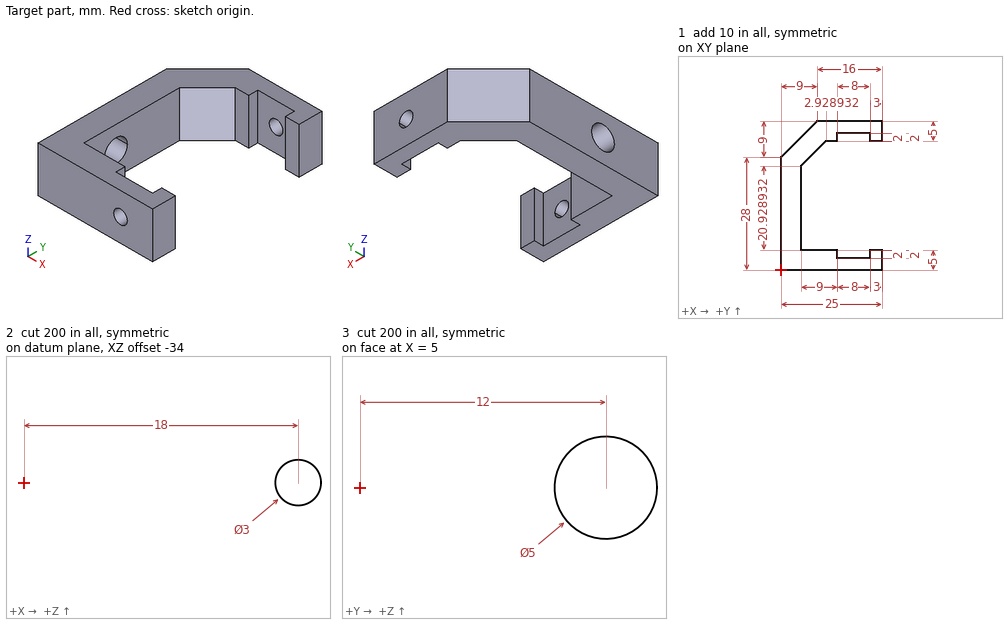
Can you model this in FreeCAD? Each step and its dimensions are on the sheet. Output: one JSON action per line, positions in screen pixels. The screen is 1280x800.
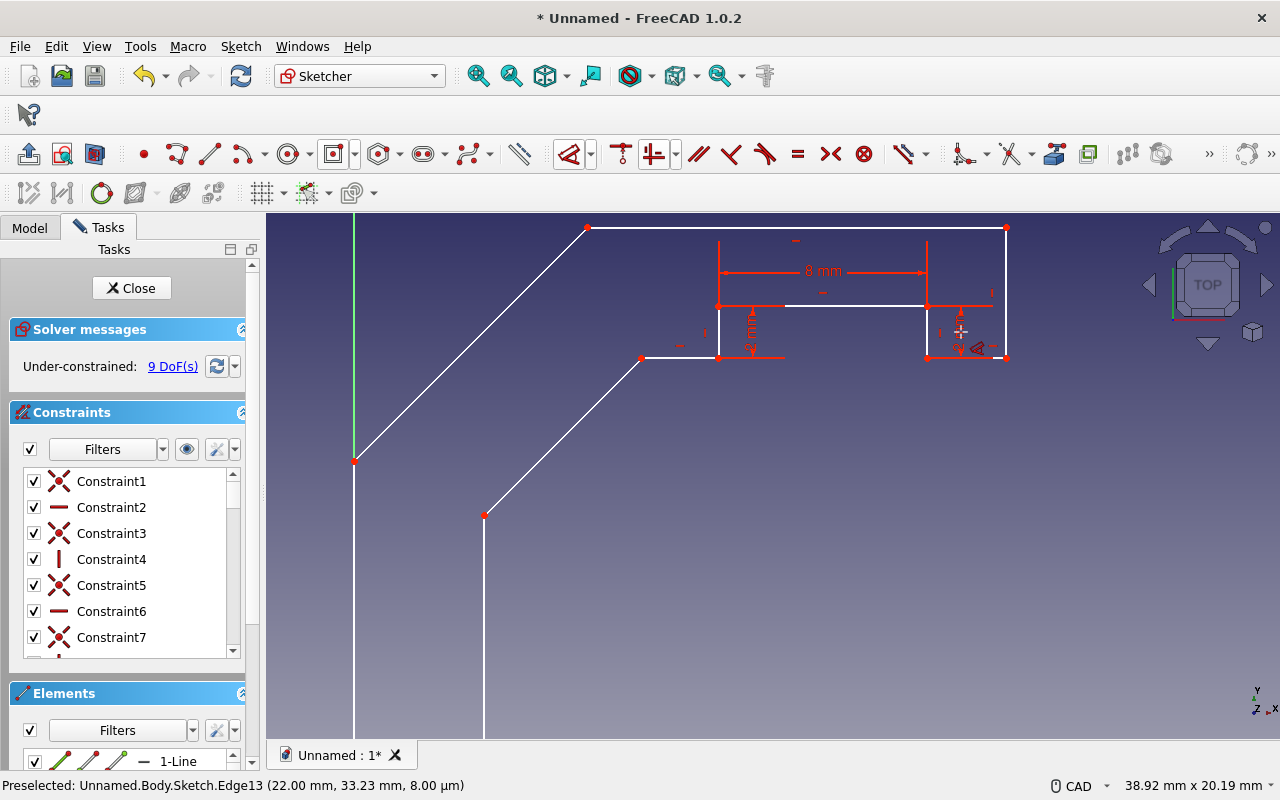
{"action": "left_click", "coordinate": [951, 358]}
{"action": "left_click", "coordinate": [967, 392]}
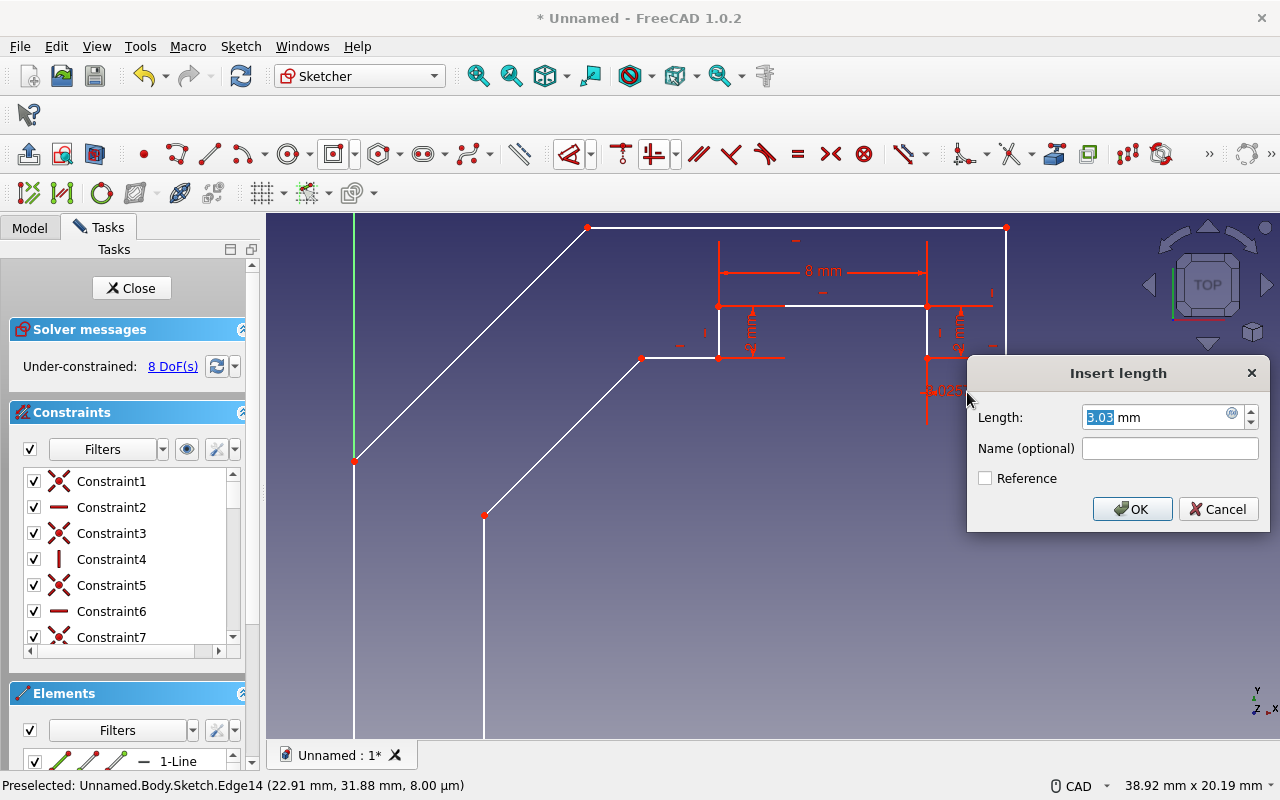
{"action": "type", "text": "3"}
{"action": "key", "text": "Return"}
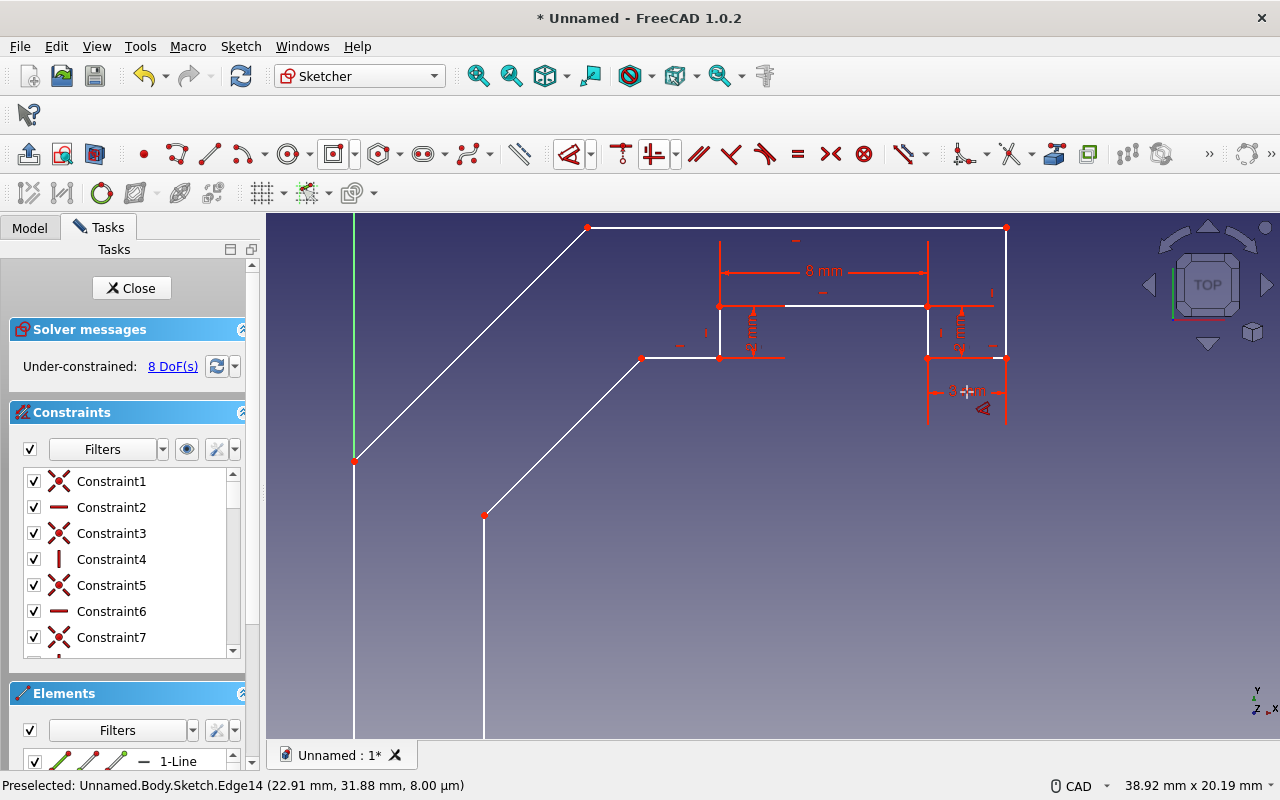
{"action": "left_click", "coordinate": [1006, 319]}
{"action": "left_click", "coordinate": [1040, 300]}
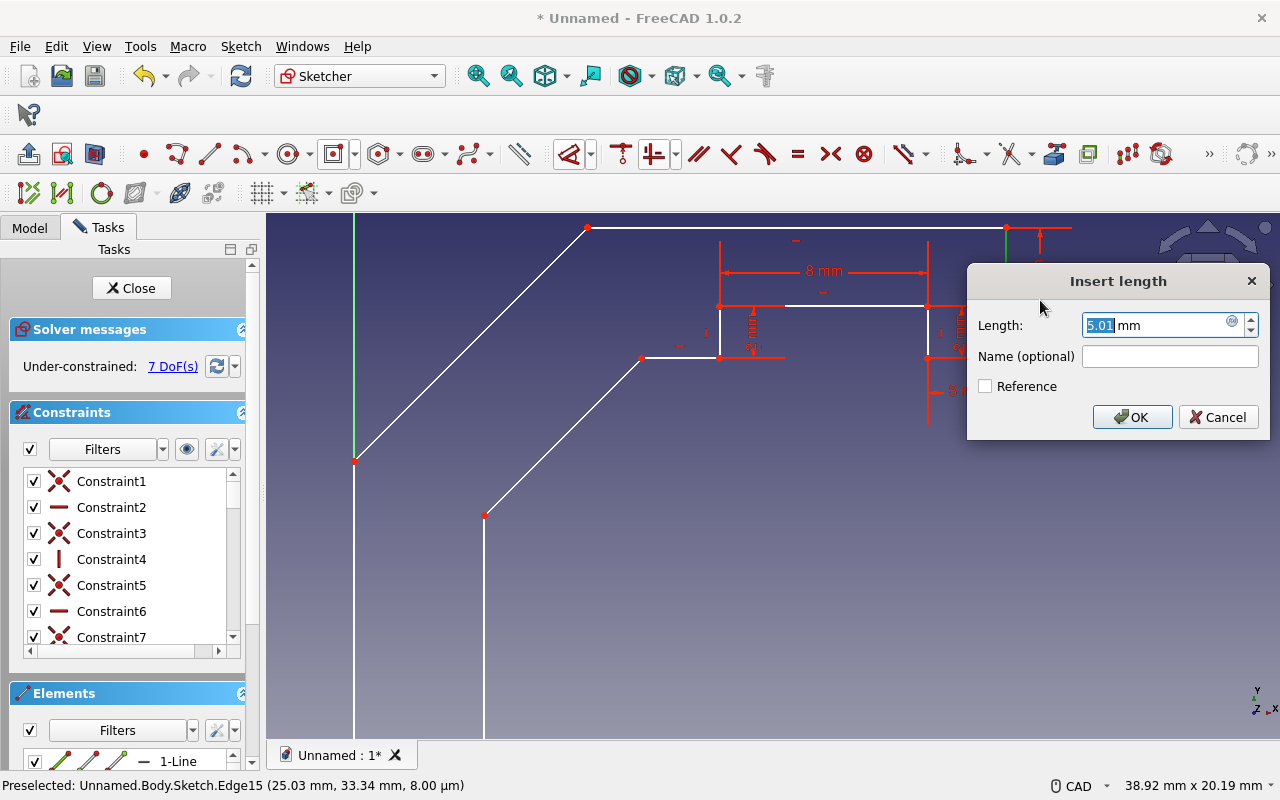
{"action": "type", "text": "5"}
{"action": "key", "text": "Return"}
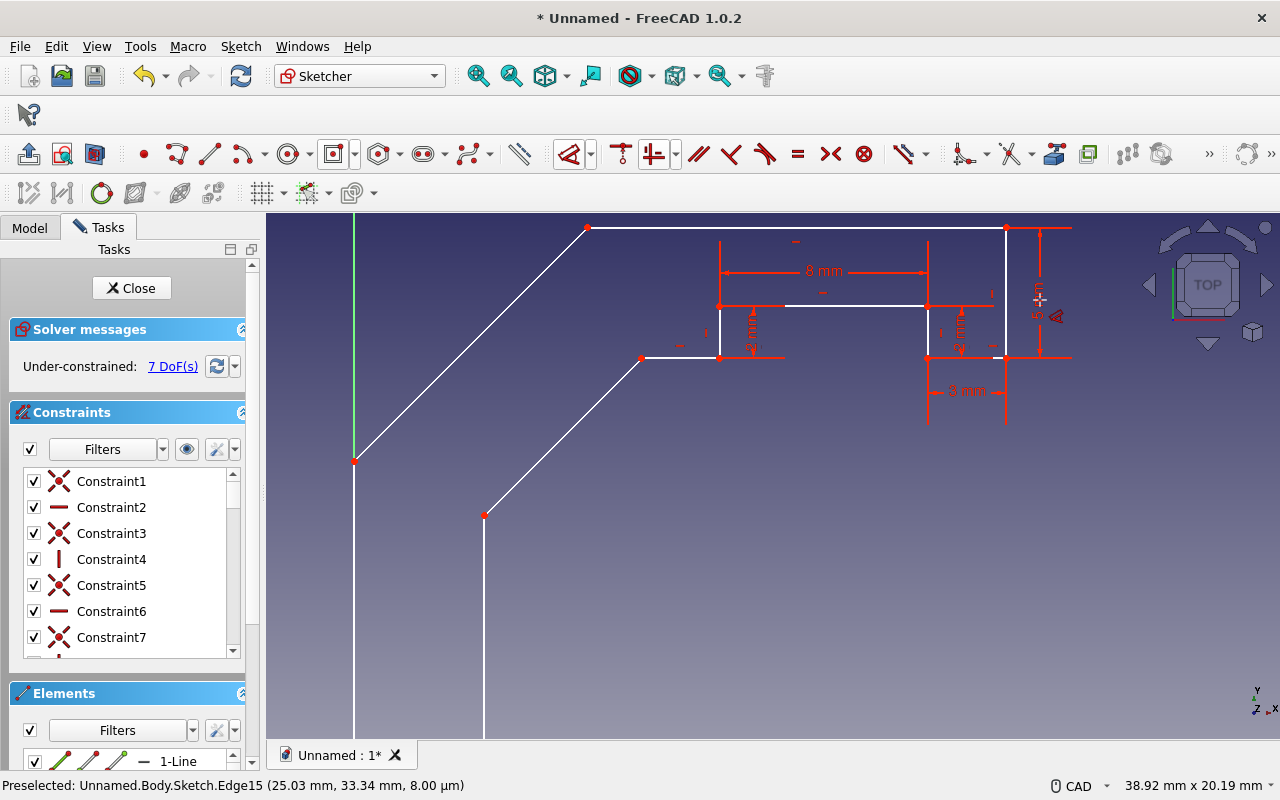
{"action": "scroll", "coordinate": [719, 342], "scroll_direction": "down", "scroll_amount": 5}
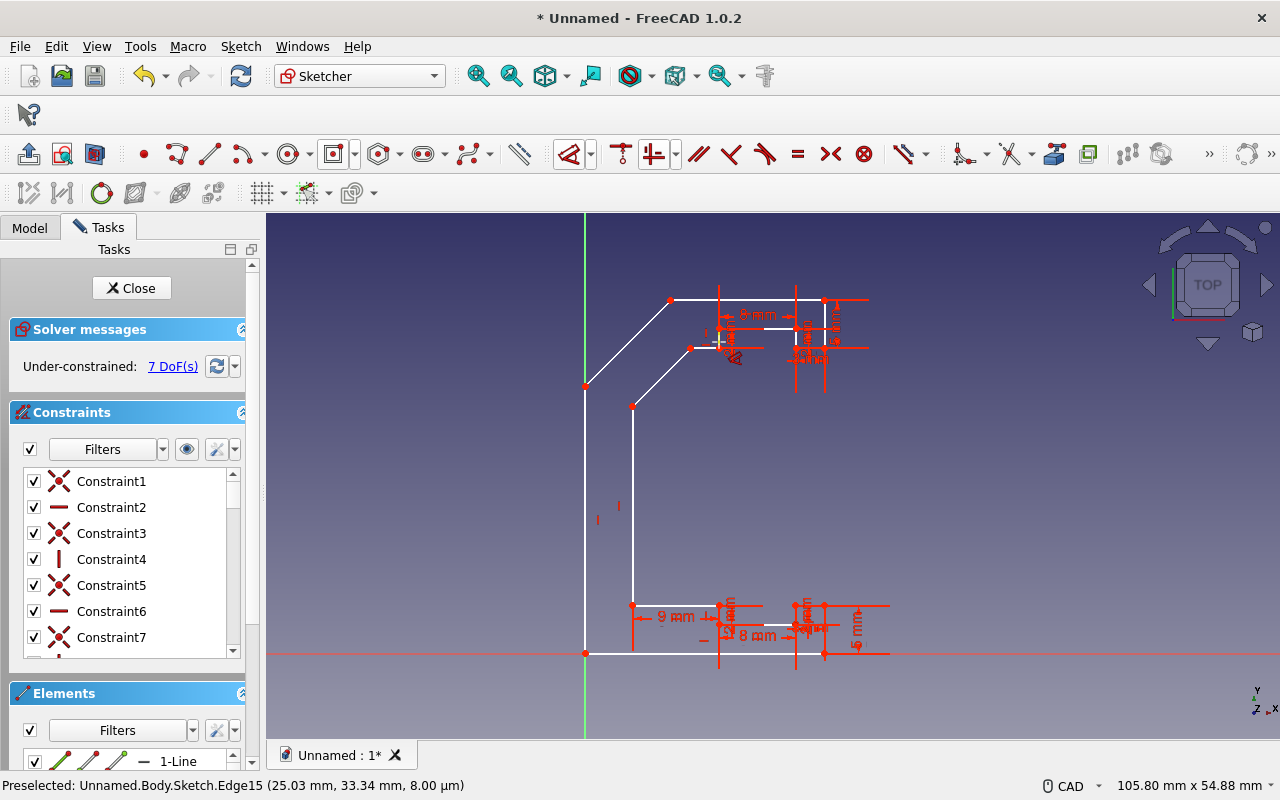
{"action": "left_click", "coordinate": [657, 654]}
{"action": "left_click", "coordinate": [705, 688]}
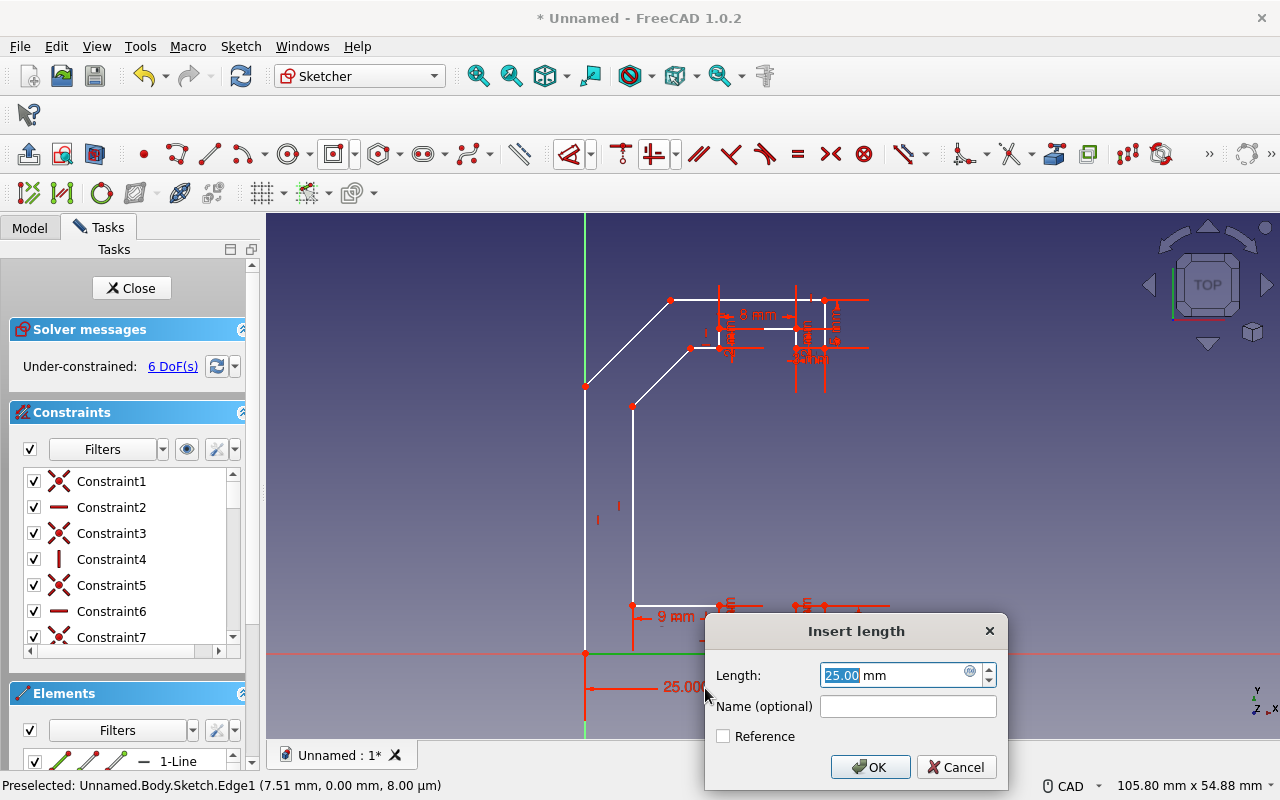
{"action": "type", "text": "25"}
{"action": "key", "text": "Return"}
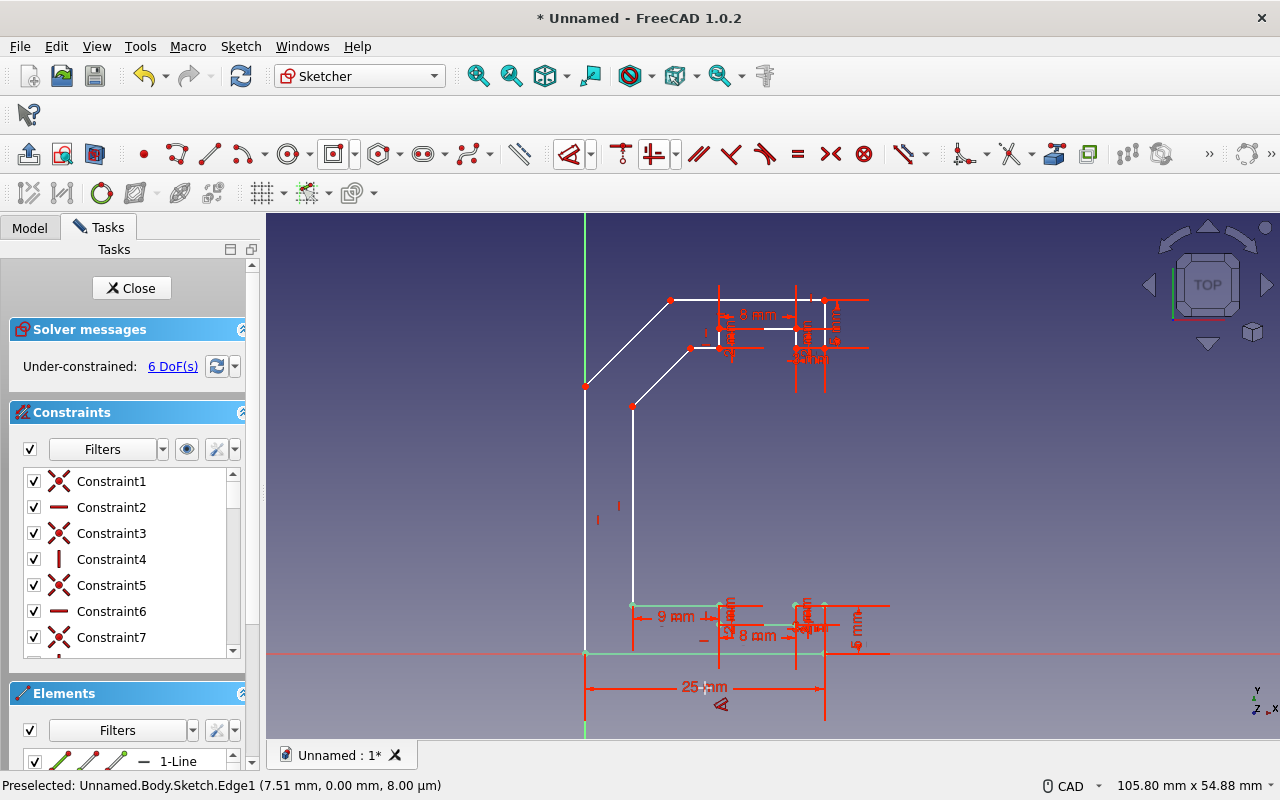
{"action": "left_click", "coordinate": [779, 300]}
{"action": "left_click", "coordinate": [748, 266]}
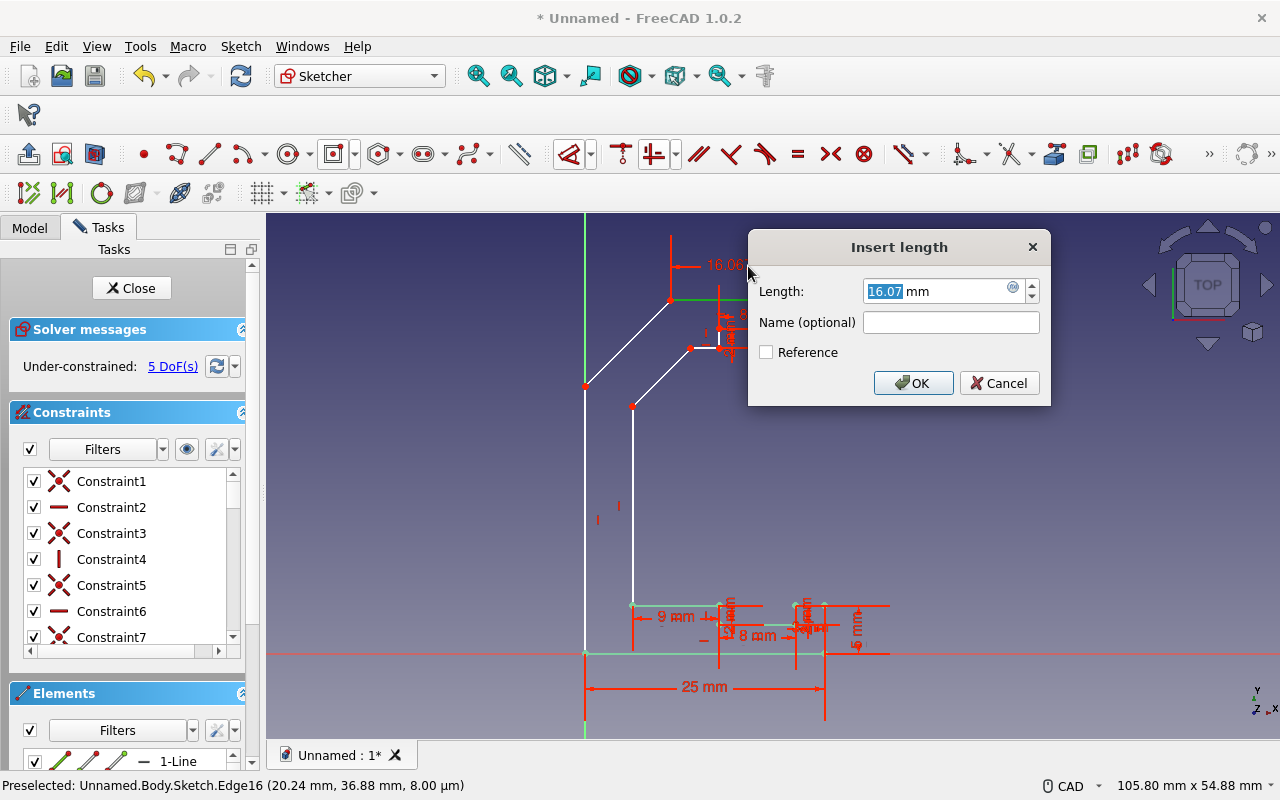
{"action": "type", "text": "16"}
{"action": "key", "text": "Return"}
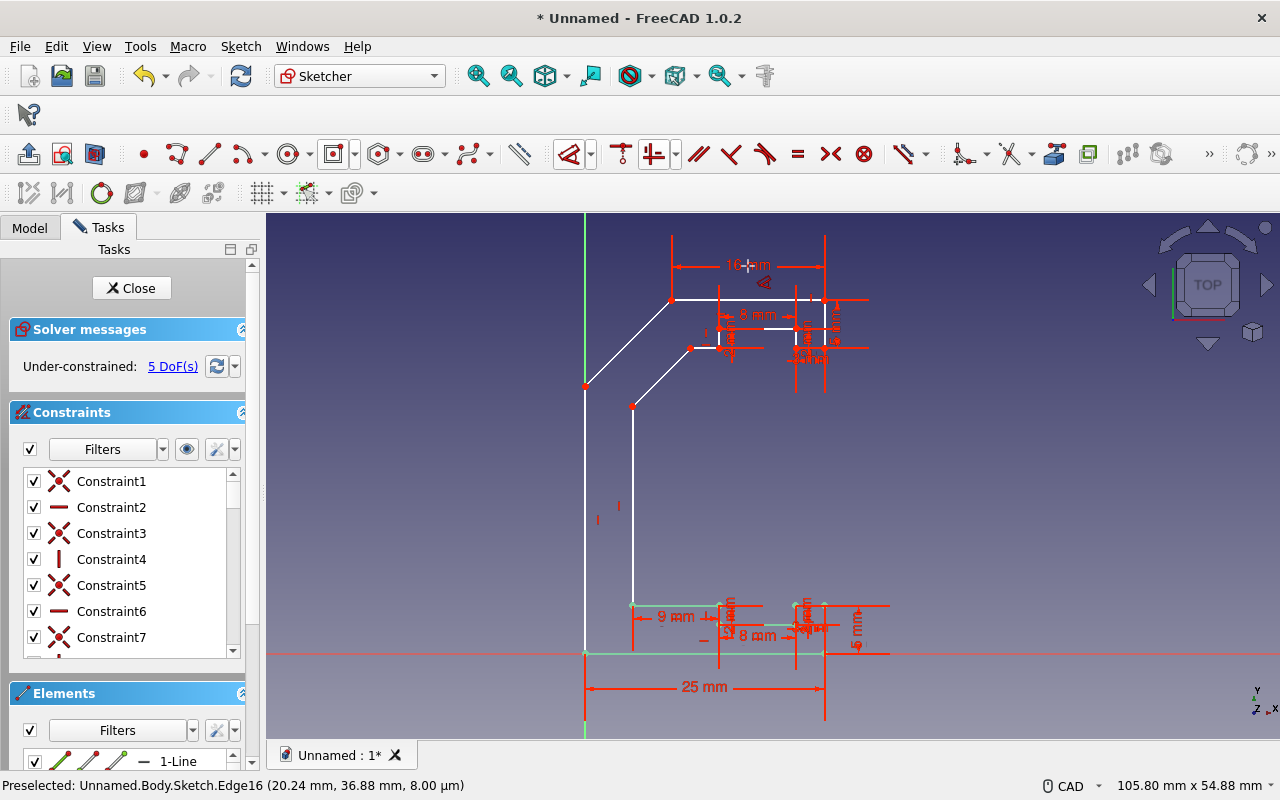
{"action": "left_click", "coordinate": [585, 466]}
{"action": "left_click", "coordinate": [551, 520]}